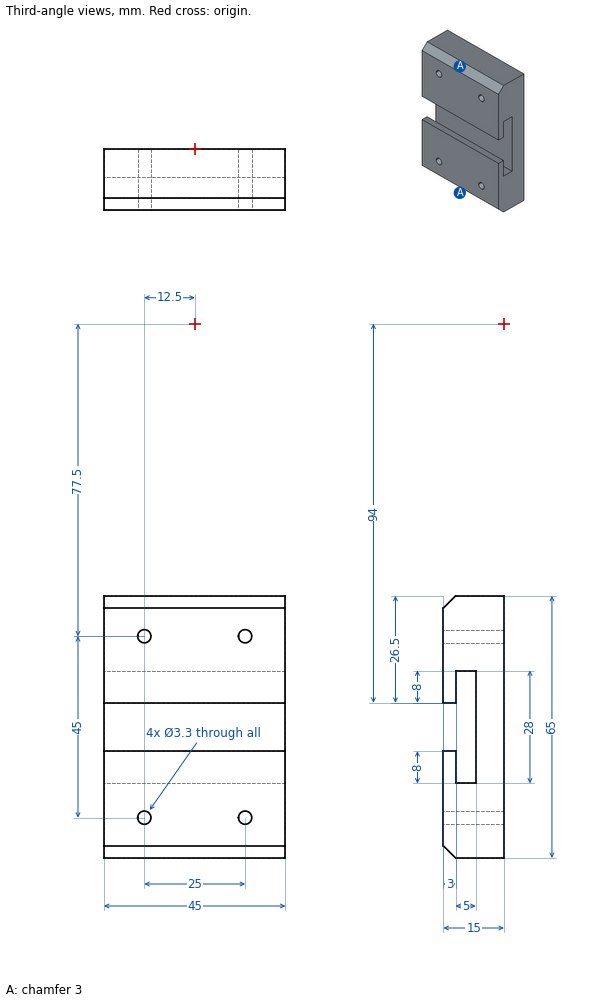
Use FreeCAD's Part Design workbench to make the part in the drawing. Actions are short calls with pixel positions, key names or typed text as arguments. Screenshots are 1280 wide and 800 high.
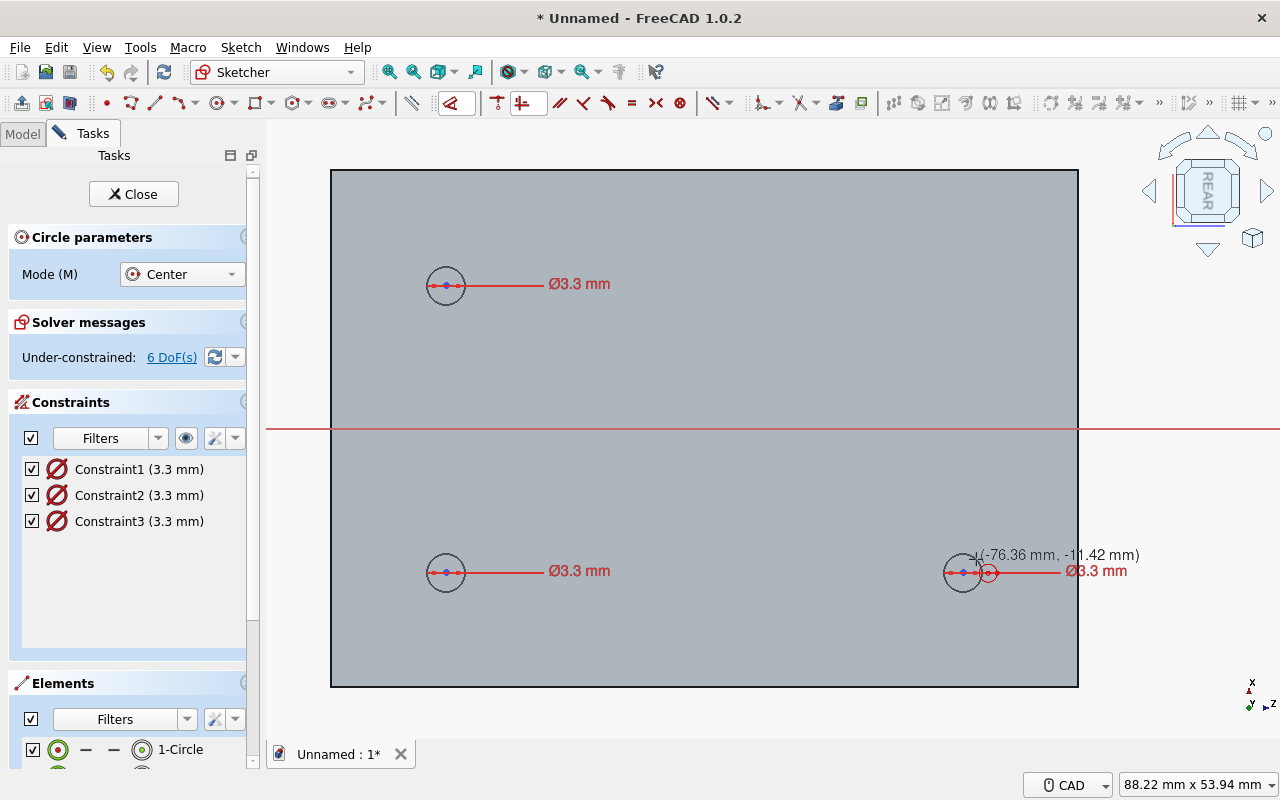
click(963, 285)
move(976, 272)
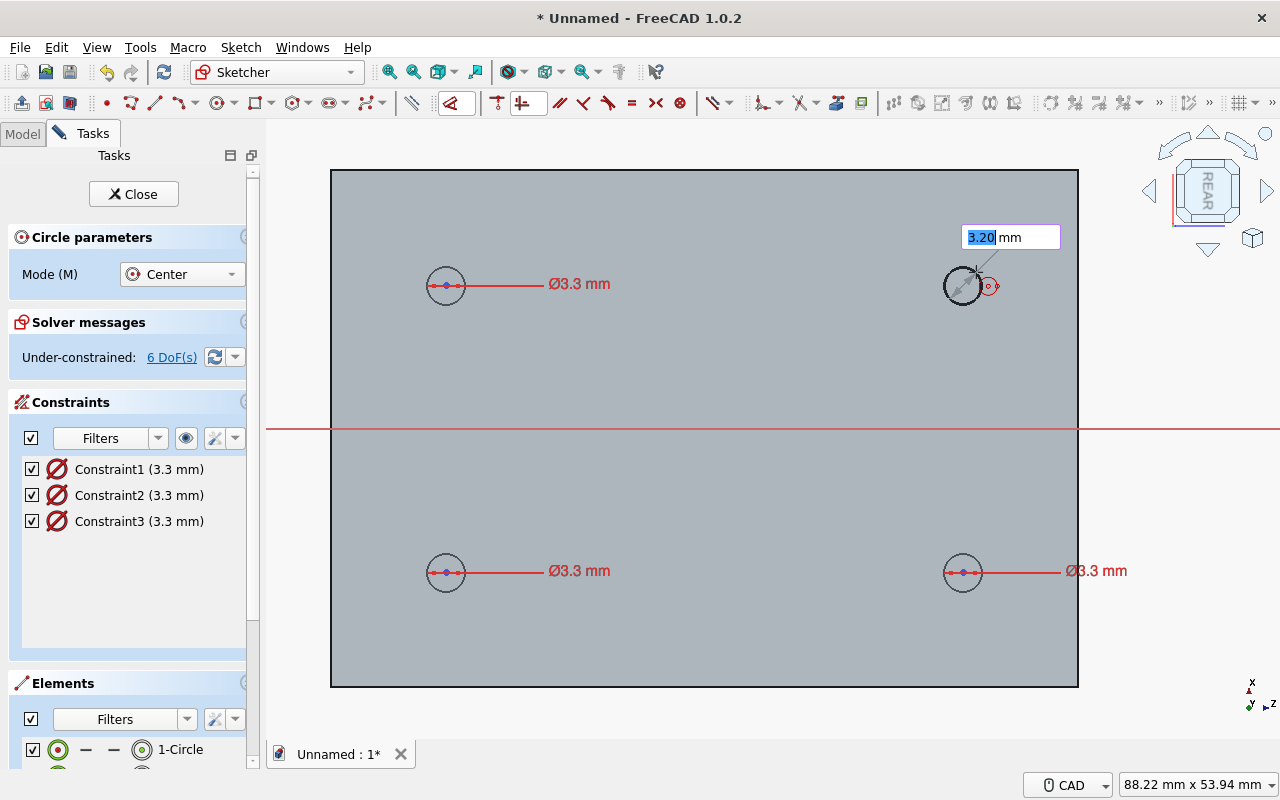
text(3.3)
key(Return)
key(Escape)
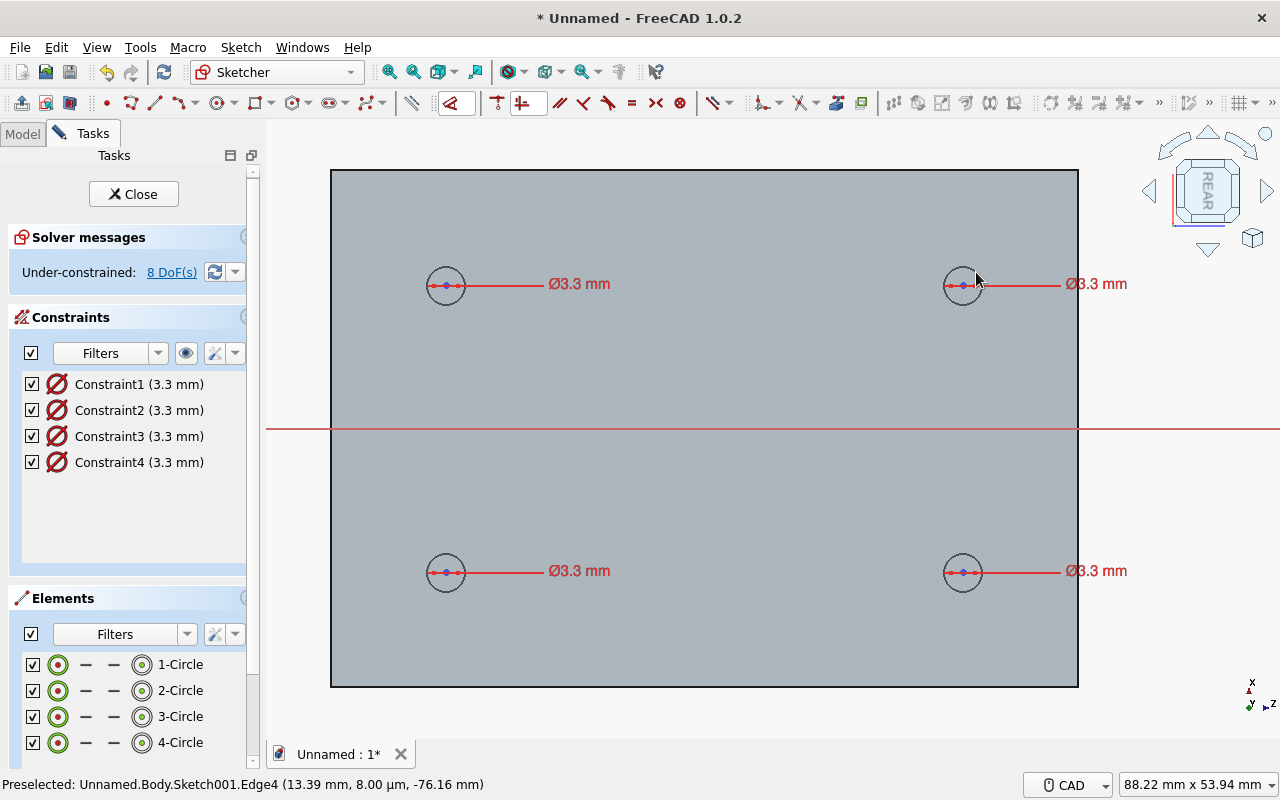
click(446, 573)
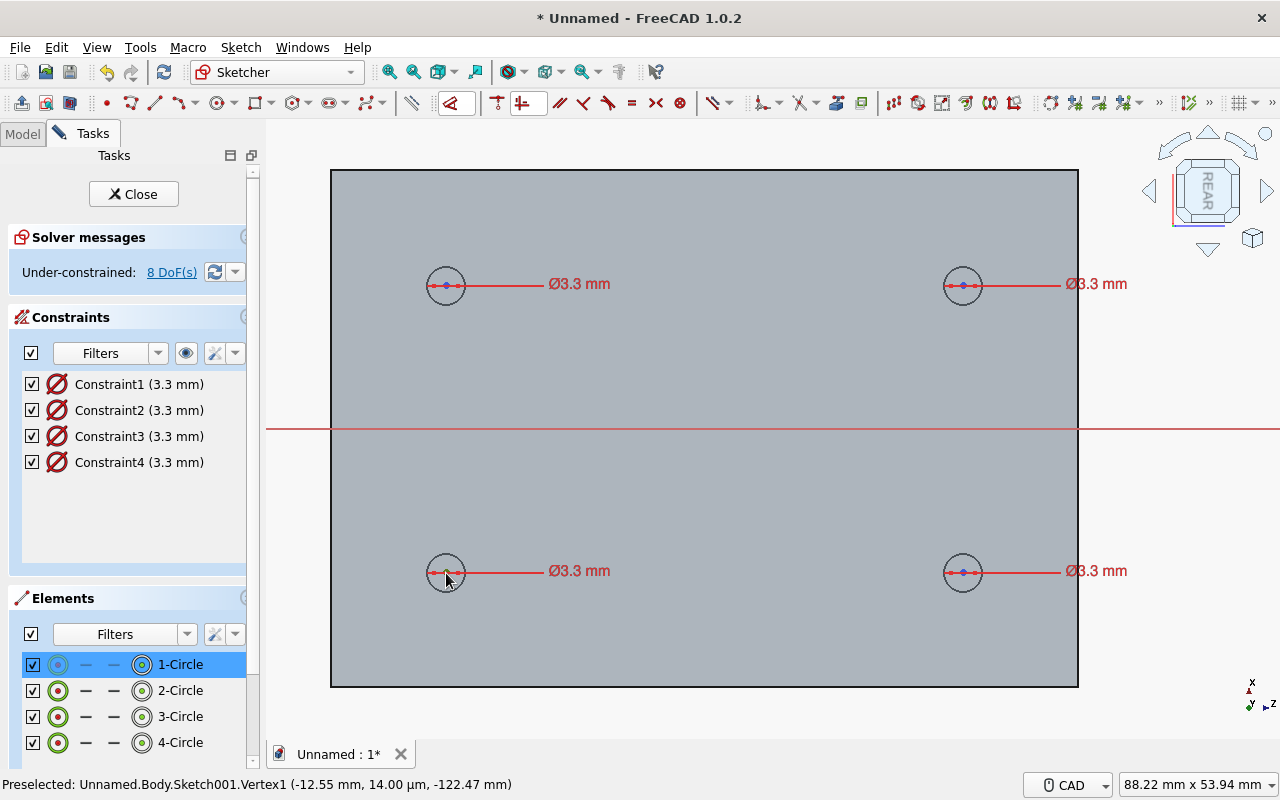
click(446, 286)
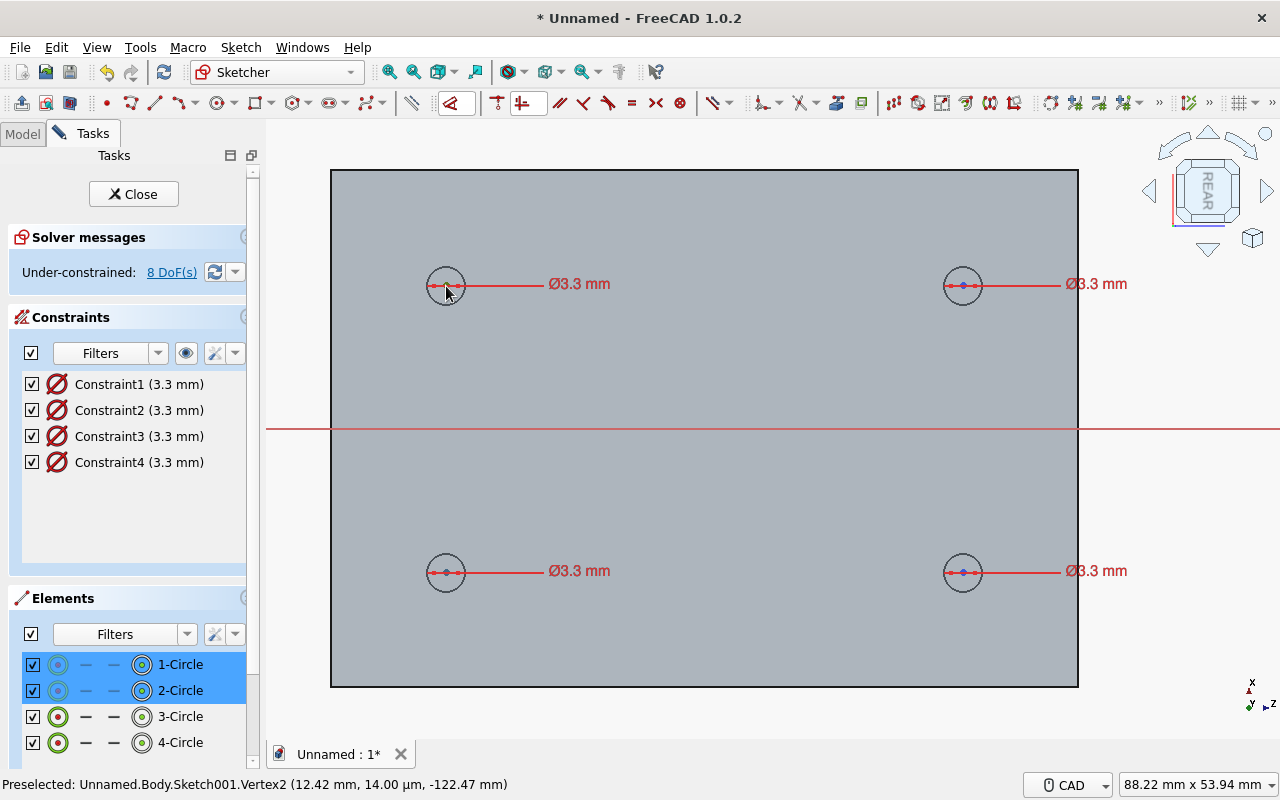
click(542, 104)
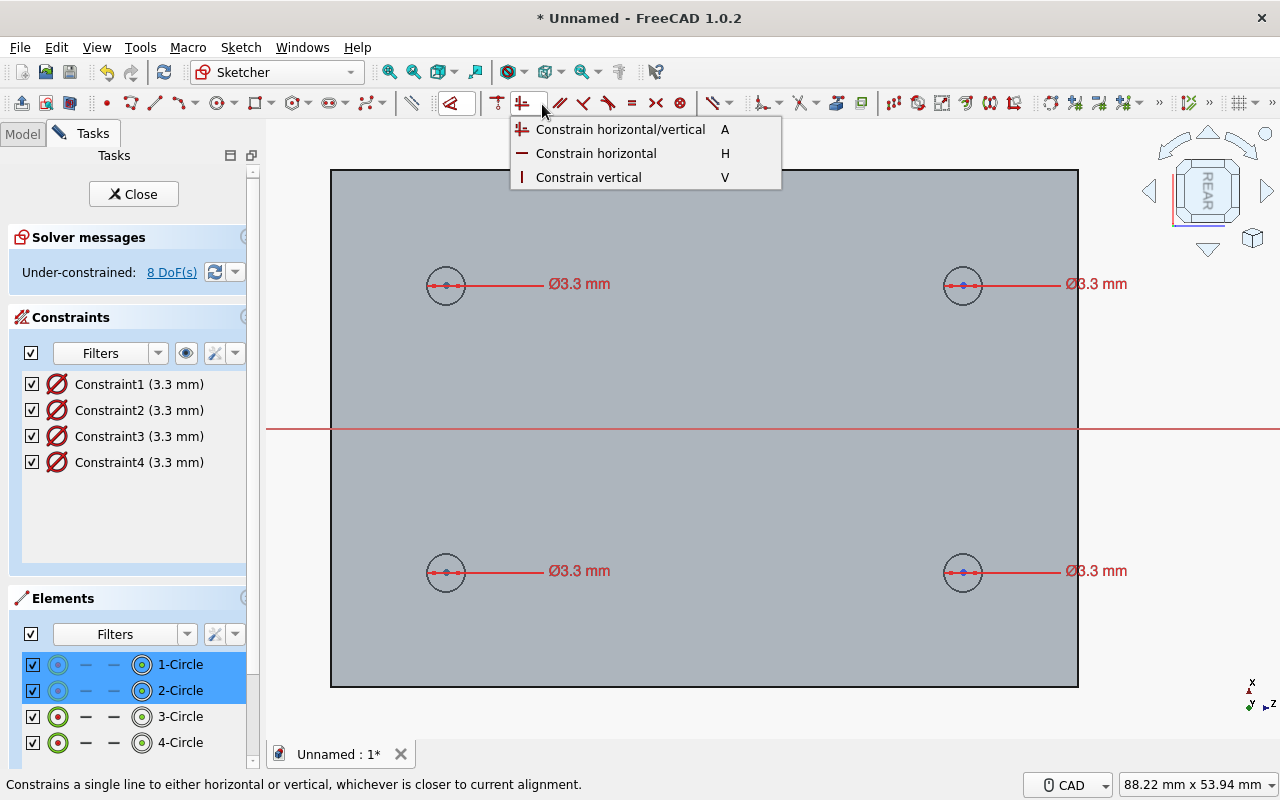
click(646, 177)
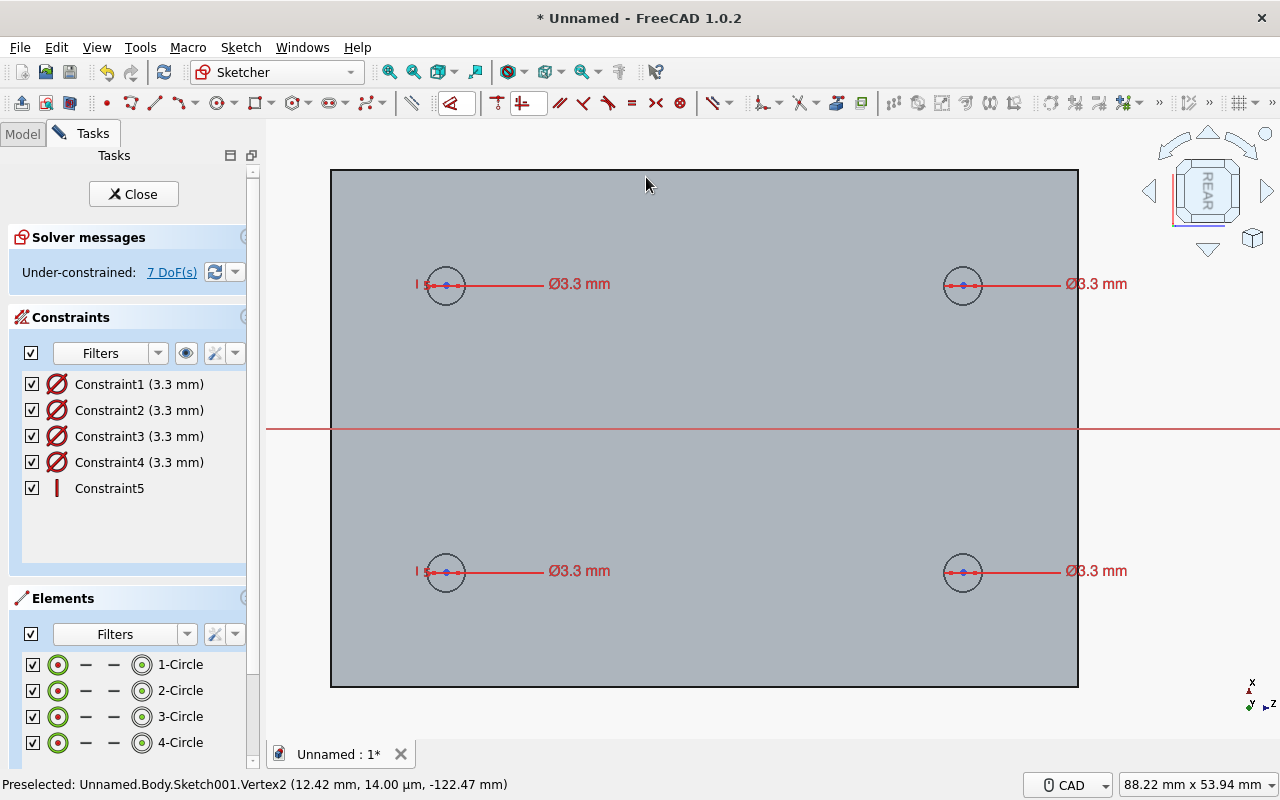
click(446, 573)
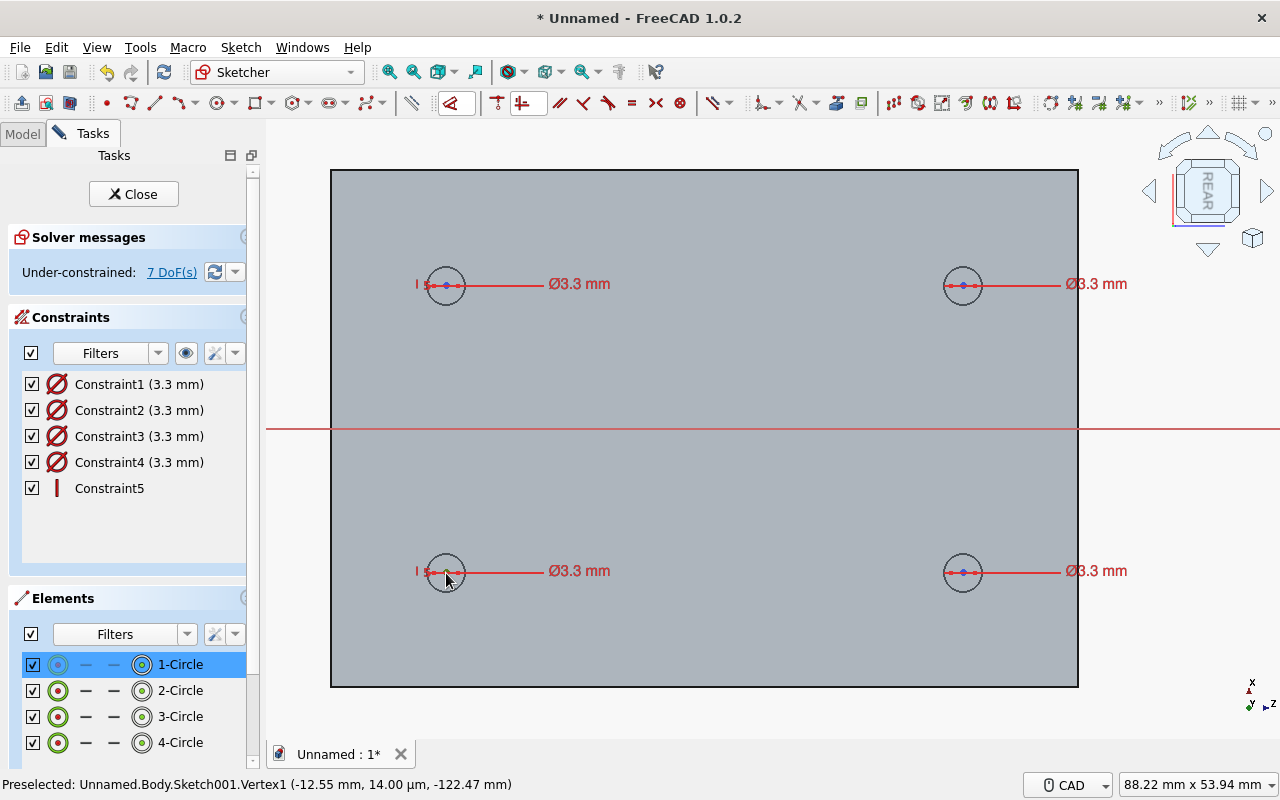
click(963, 573)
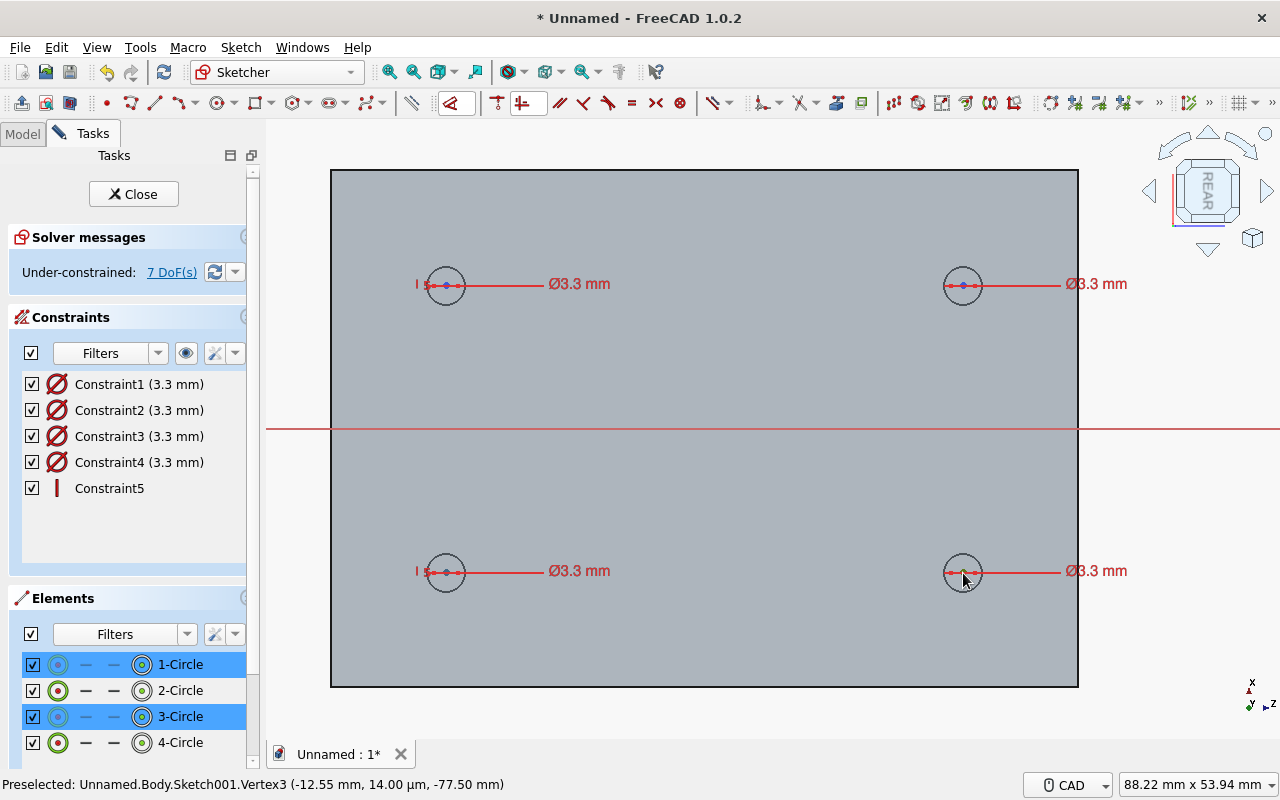
key(h)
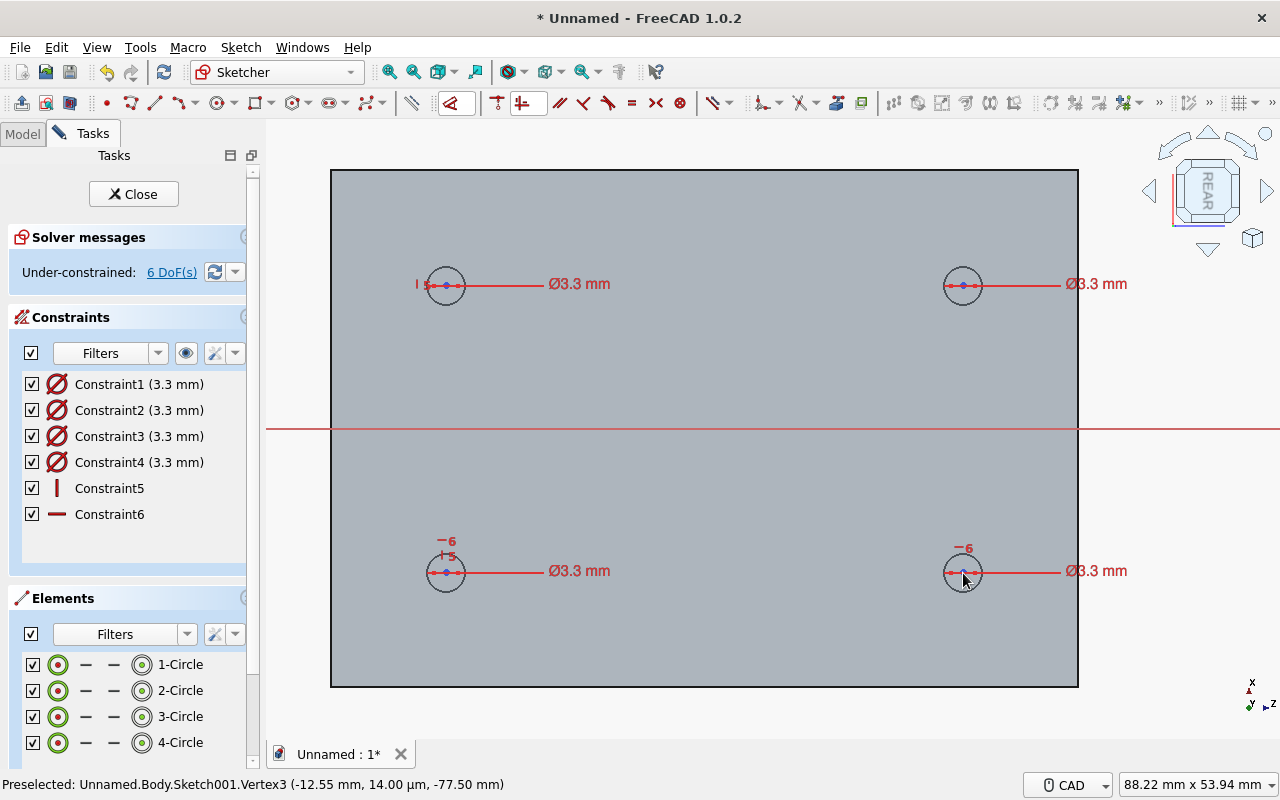
click(963, 573)